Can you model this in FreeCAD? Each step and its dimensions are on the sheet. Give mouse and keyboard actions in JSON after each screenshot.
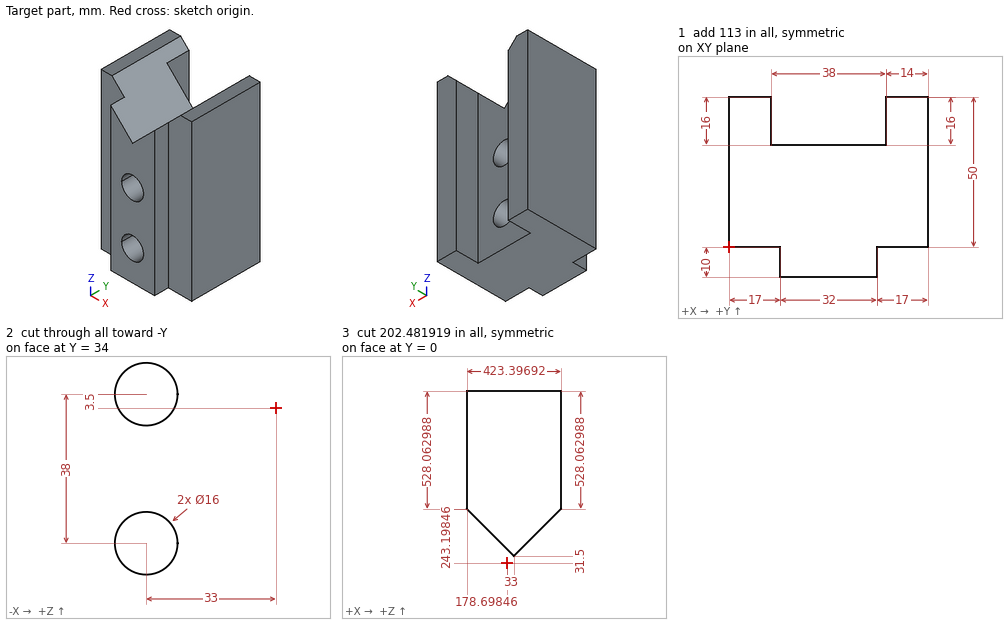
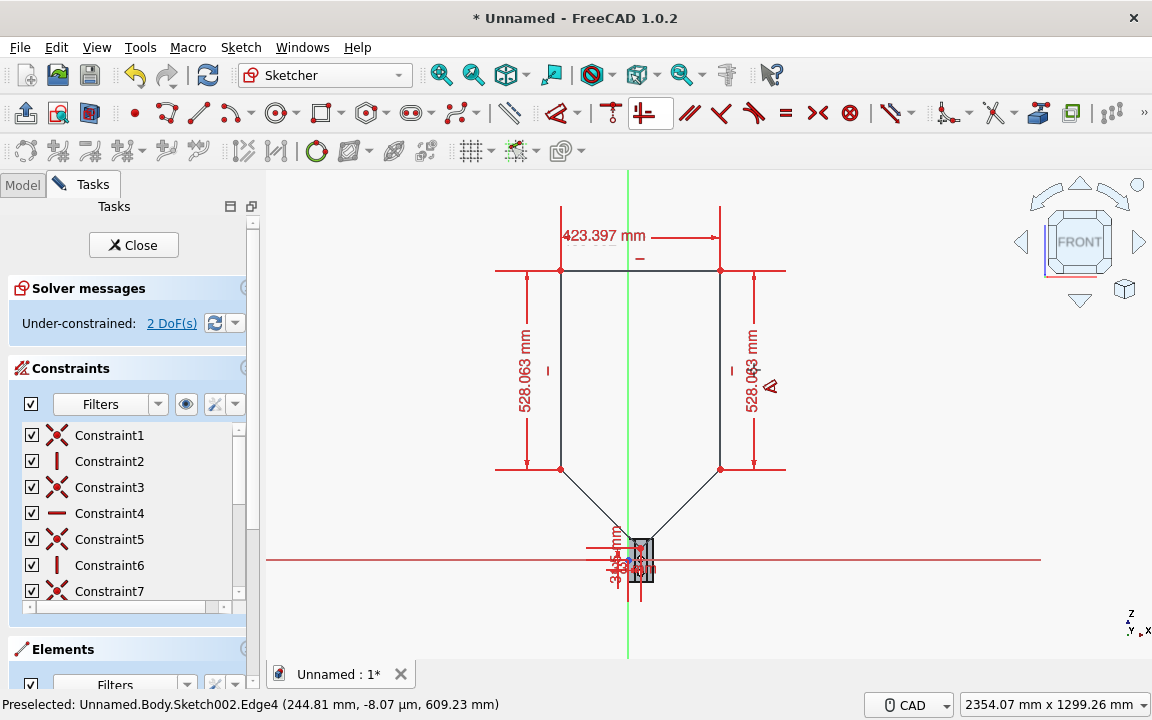
{"action": "left_click", "coordinate": [561, 470]}
{"action": "left_click", "coordinate": [595, 594]}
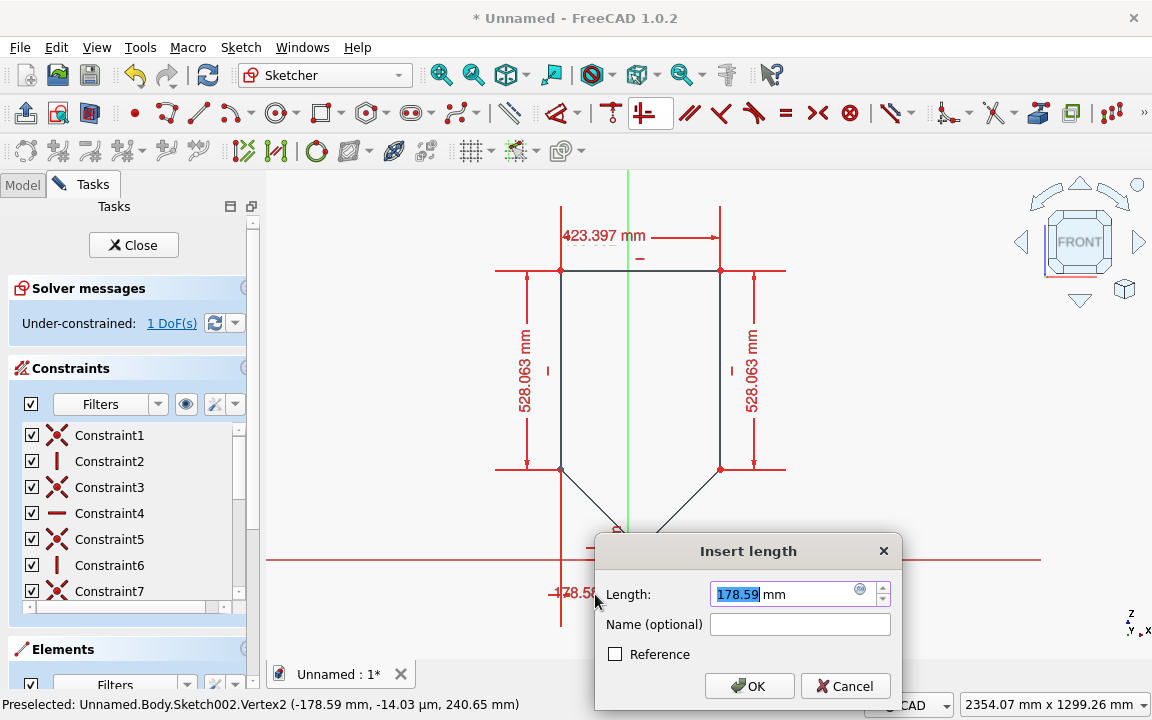
{"action": "type", "text": "178.69846"}
{"action": "key", "text": "Return"}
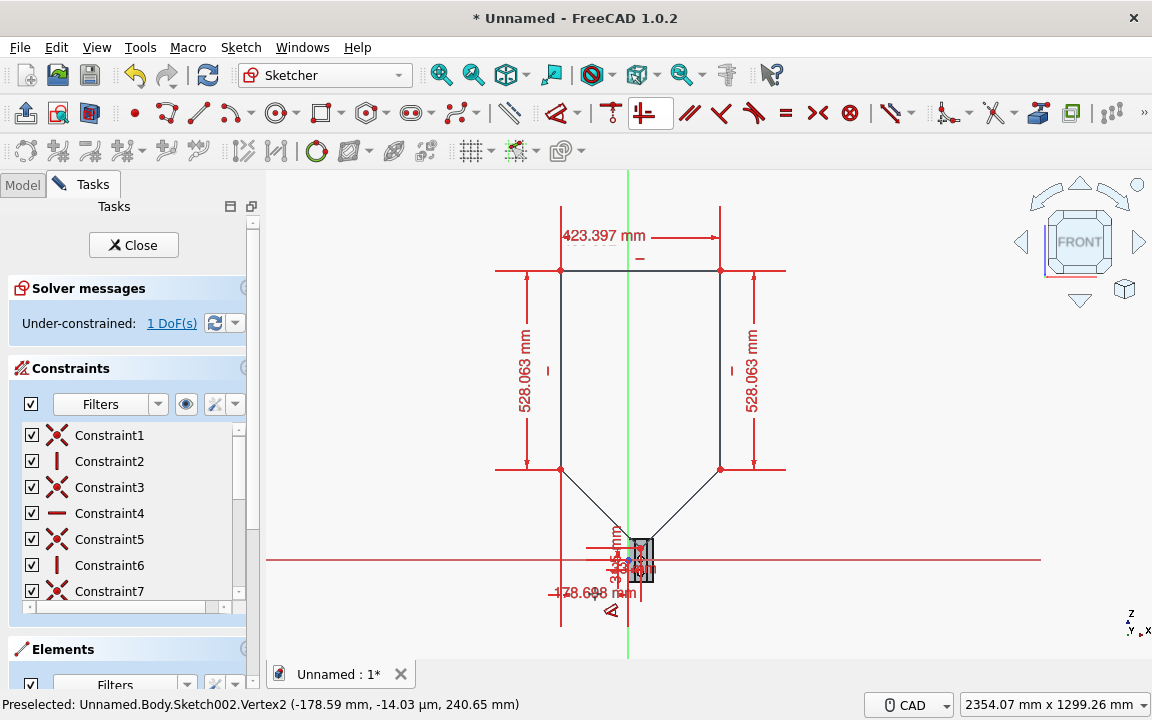
{"action": "left_click", "coordinate": [561, 470]}
{"action": "left_click", "coordinate": [527, 515]}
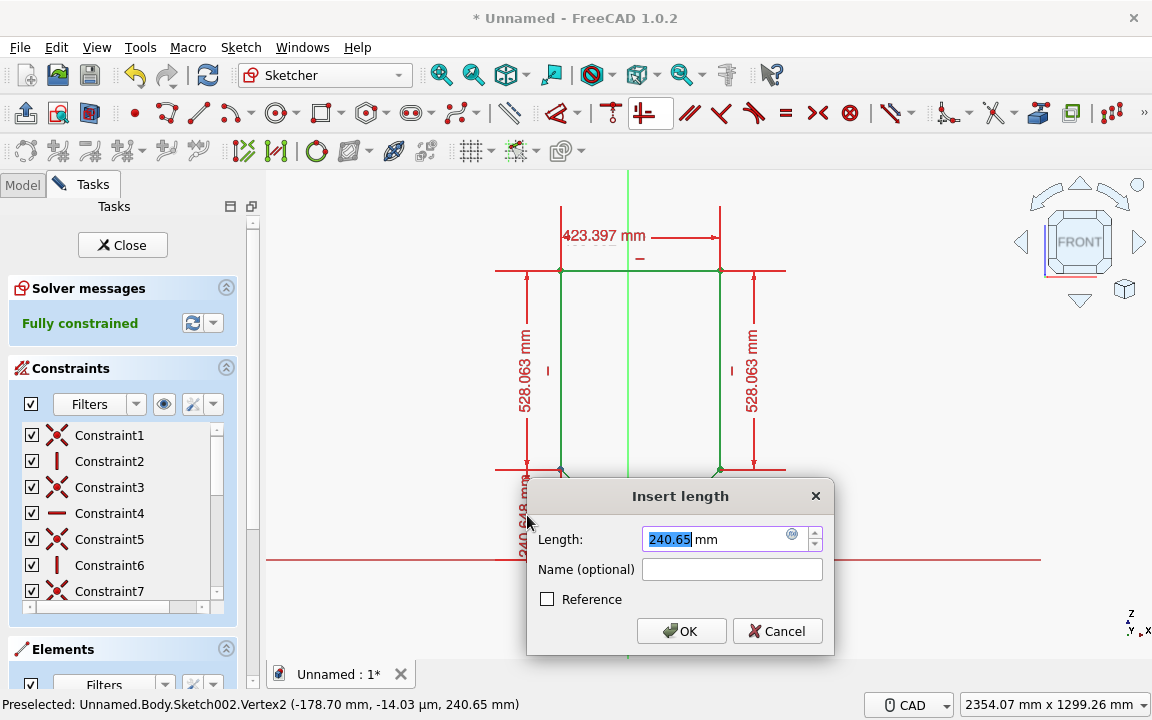
{"action": "type", "text": "243.19846"}
{"action": "key", "text": "Return"}
{"action": "key", "text": "Escape"}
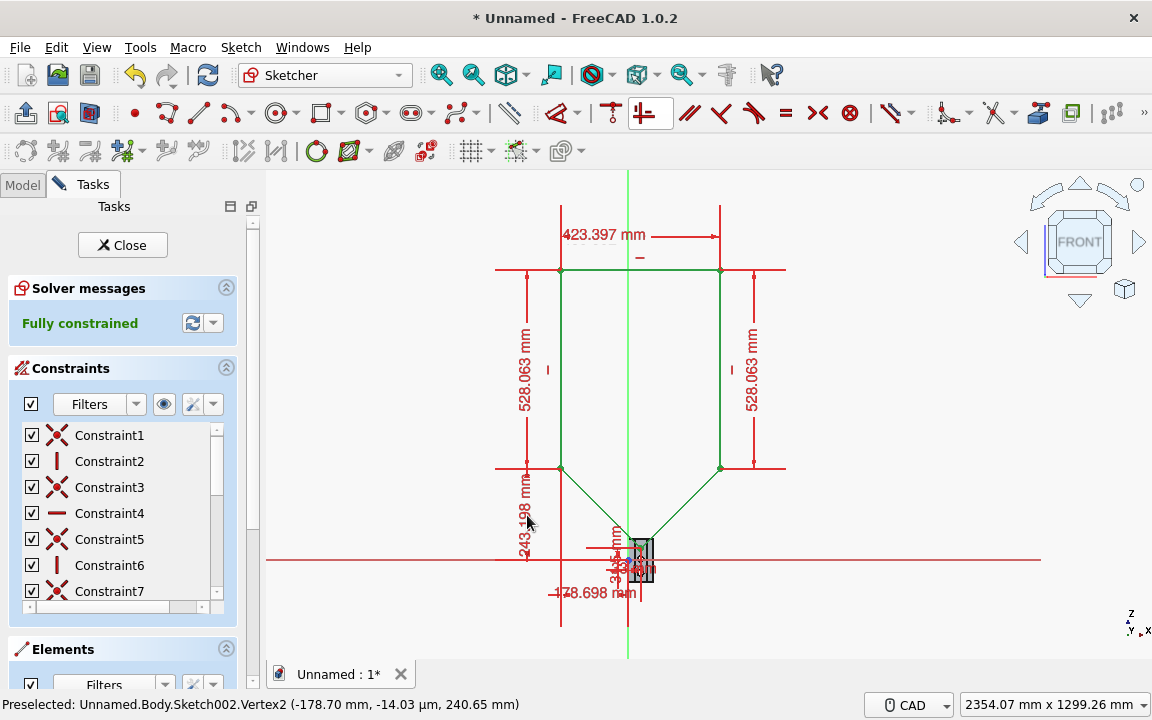
{"action": "left_click", "coordinate": [123, 245]}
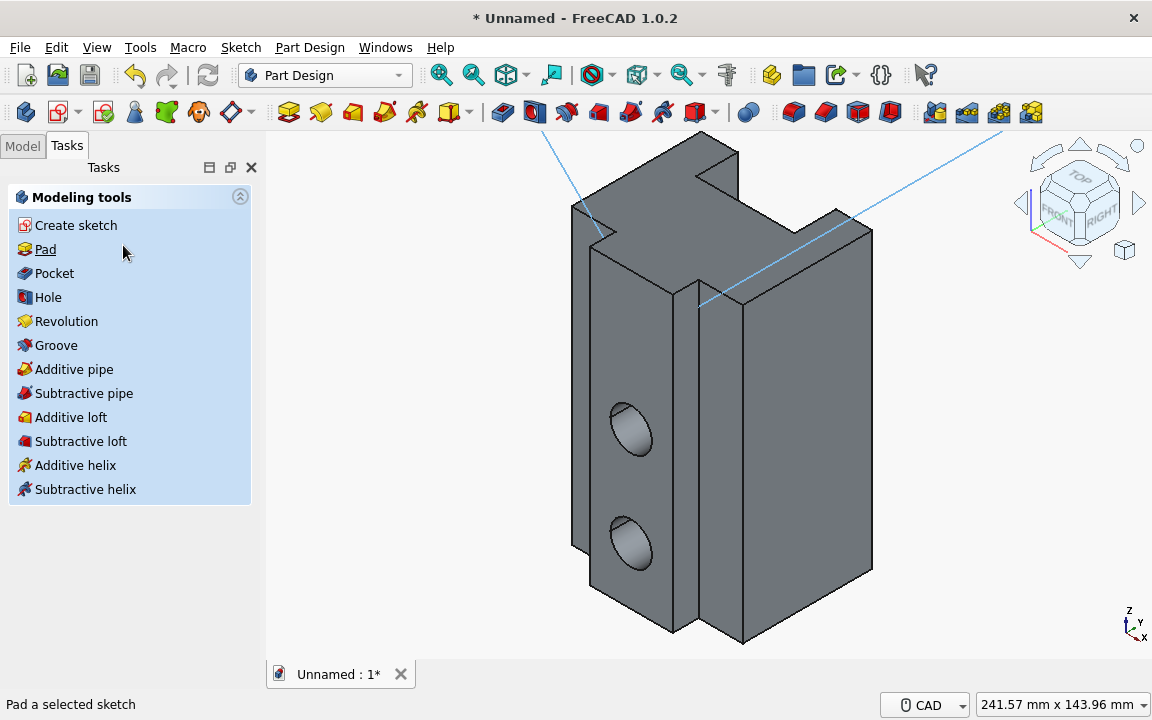
{"action": "left_click", "coordinate": [504, 112]}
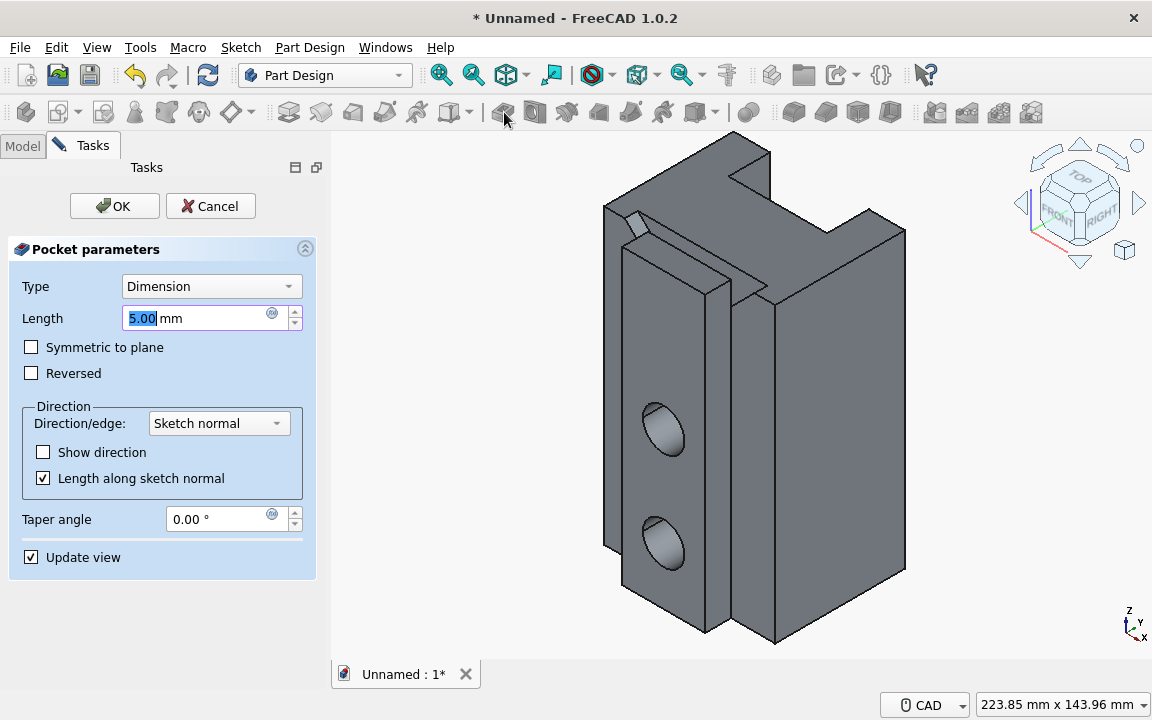
{"action": "type", "text": "202.481919"}
{"action": "key", "text": "Tab"}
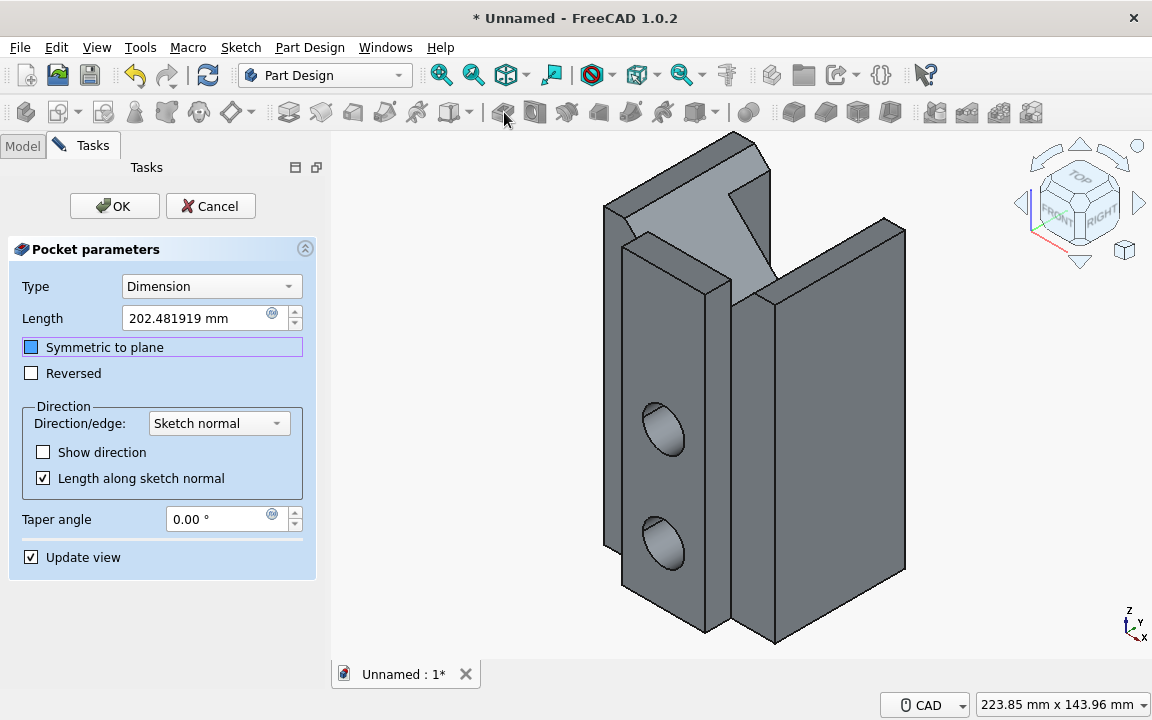
{"action": "left_click", "coordinate": [30, 347]}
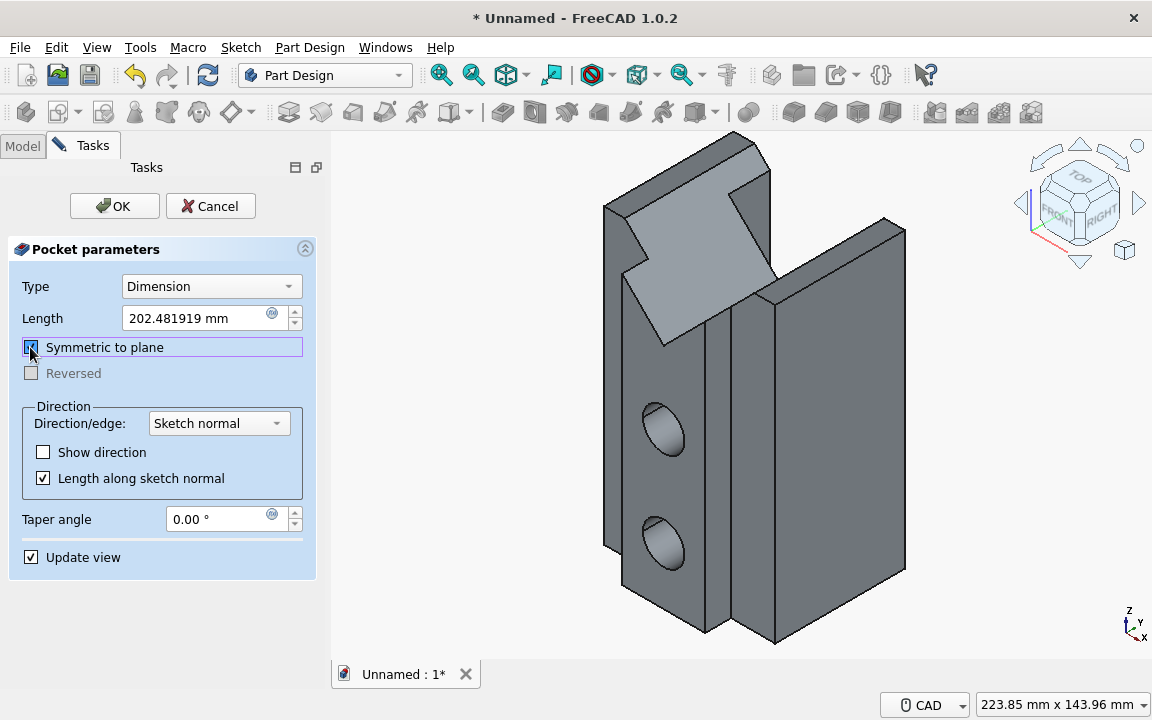
{"action": "left_click", "coordinate": [115, 206]}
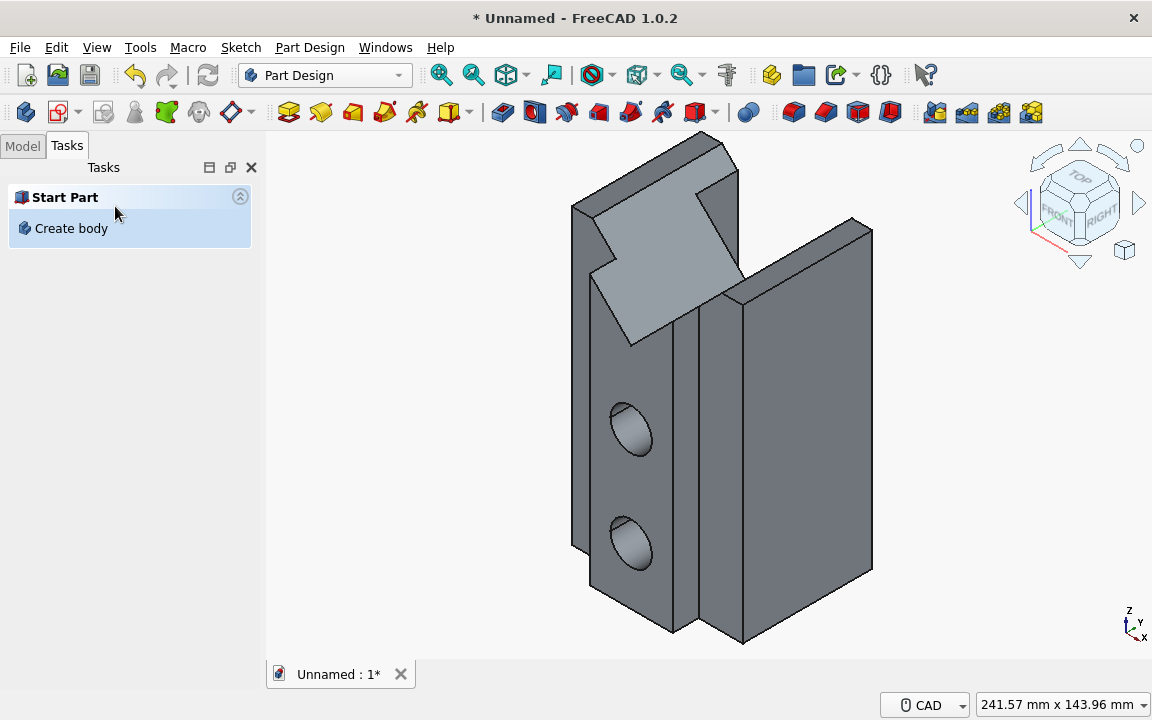
{"action": "left_click", "coordinate": [442, 76]}